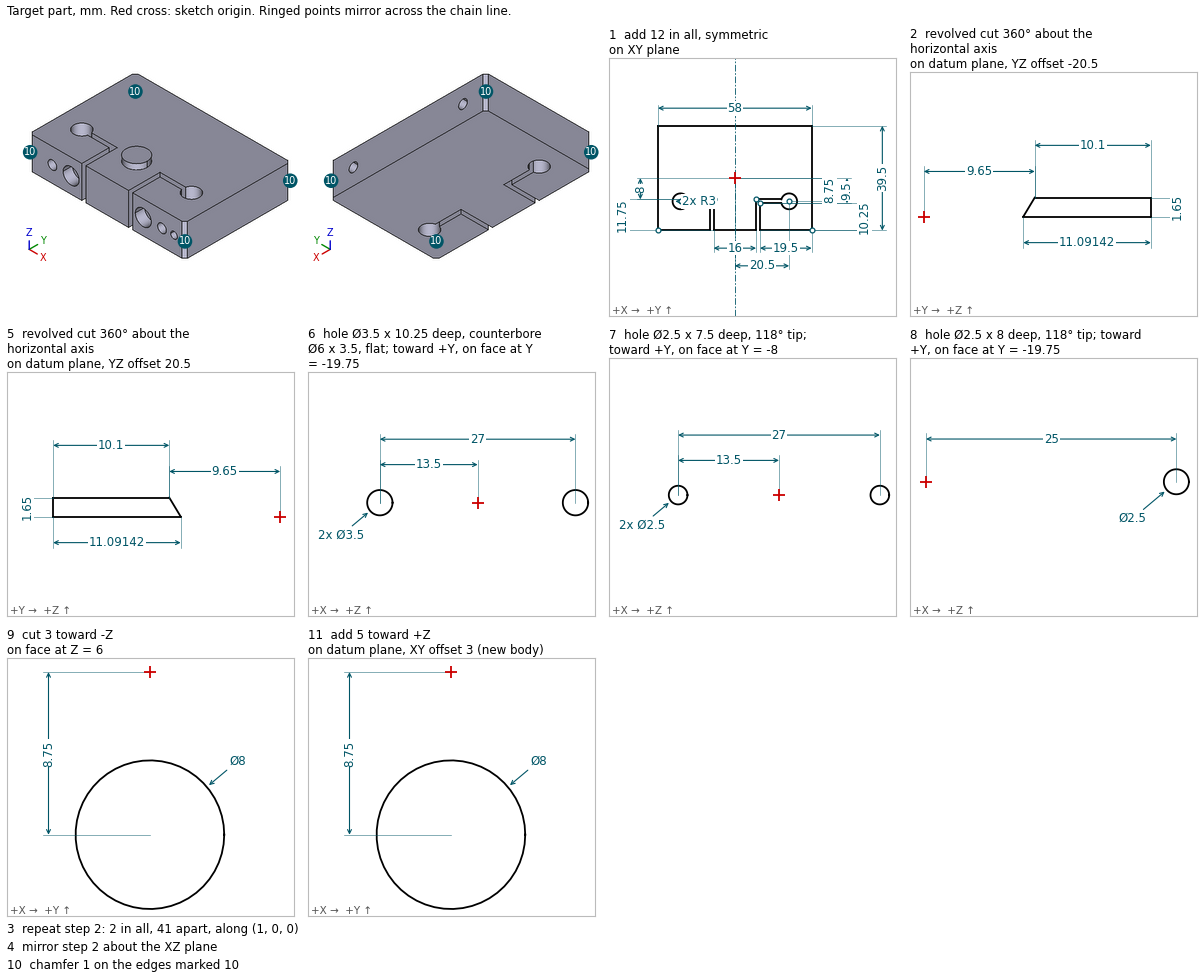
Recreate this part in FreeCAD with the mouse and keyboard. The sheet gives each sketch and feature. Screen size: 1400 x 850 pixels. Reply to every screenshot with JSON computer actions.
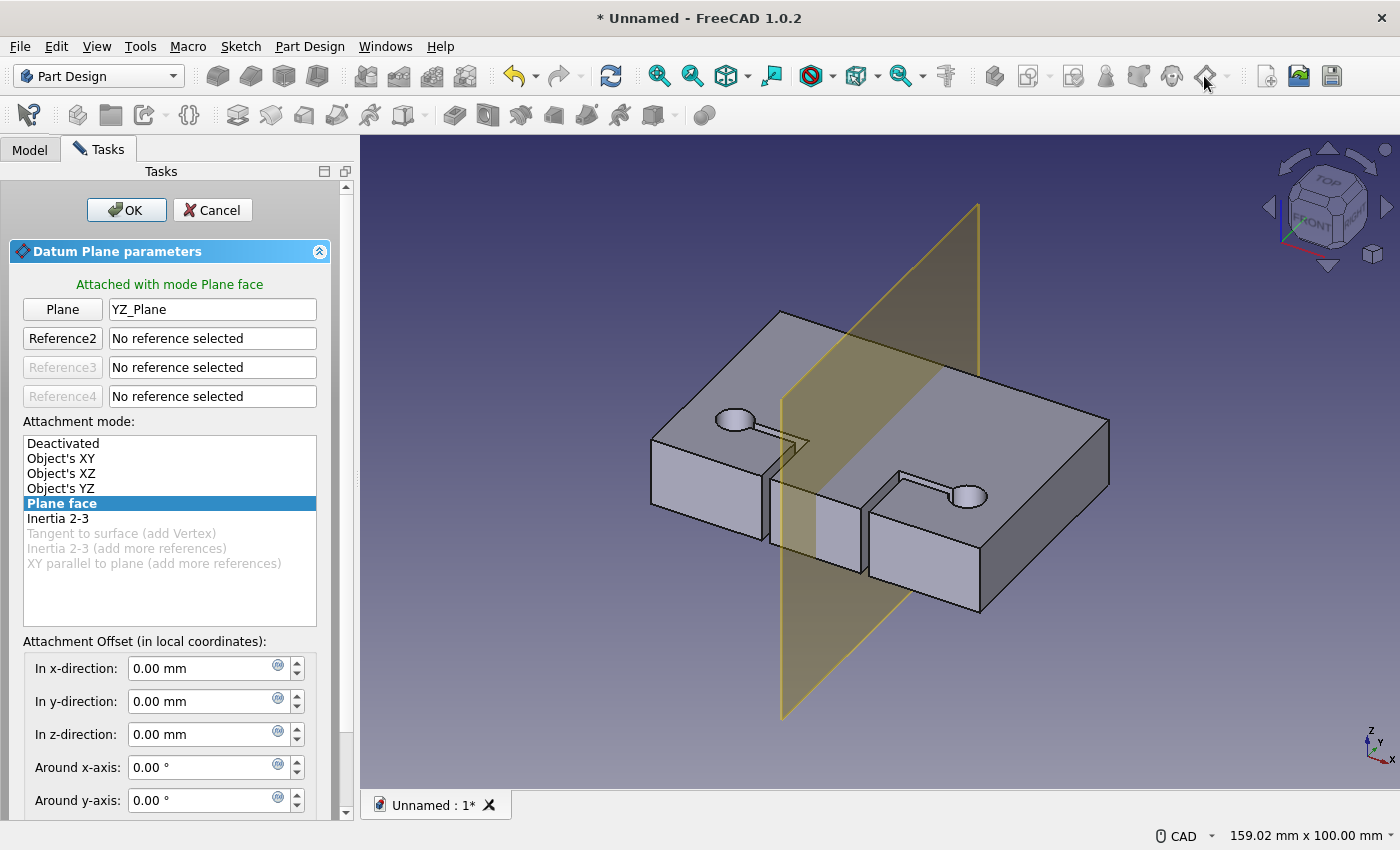
{"action": "triple_click", "coordinate": [210, 734]}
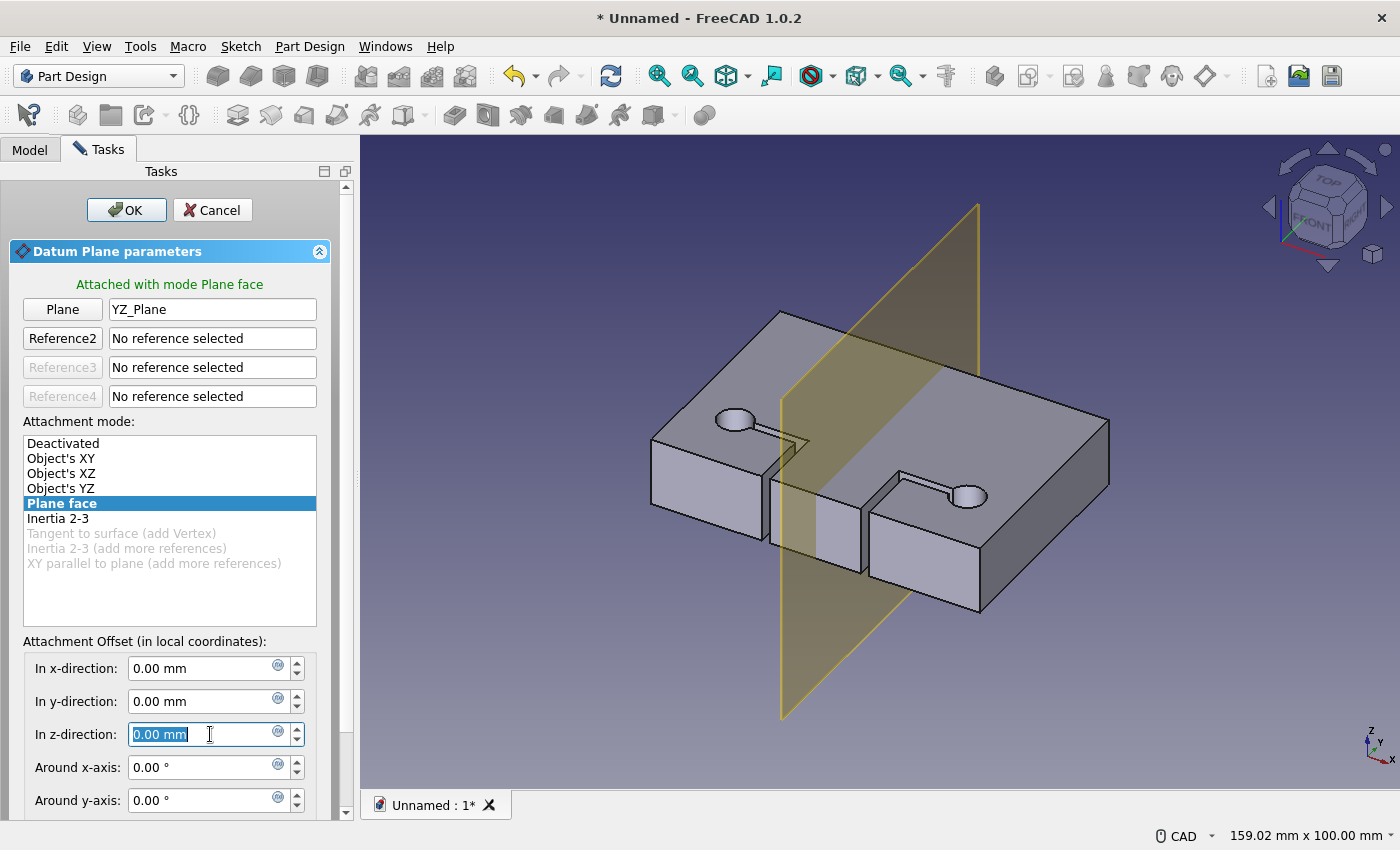
{"action": "type", "text": "-20.5"}
{"action": "key", "text": "Tab"}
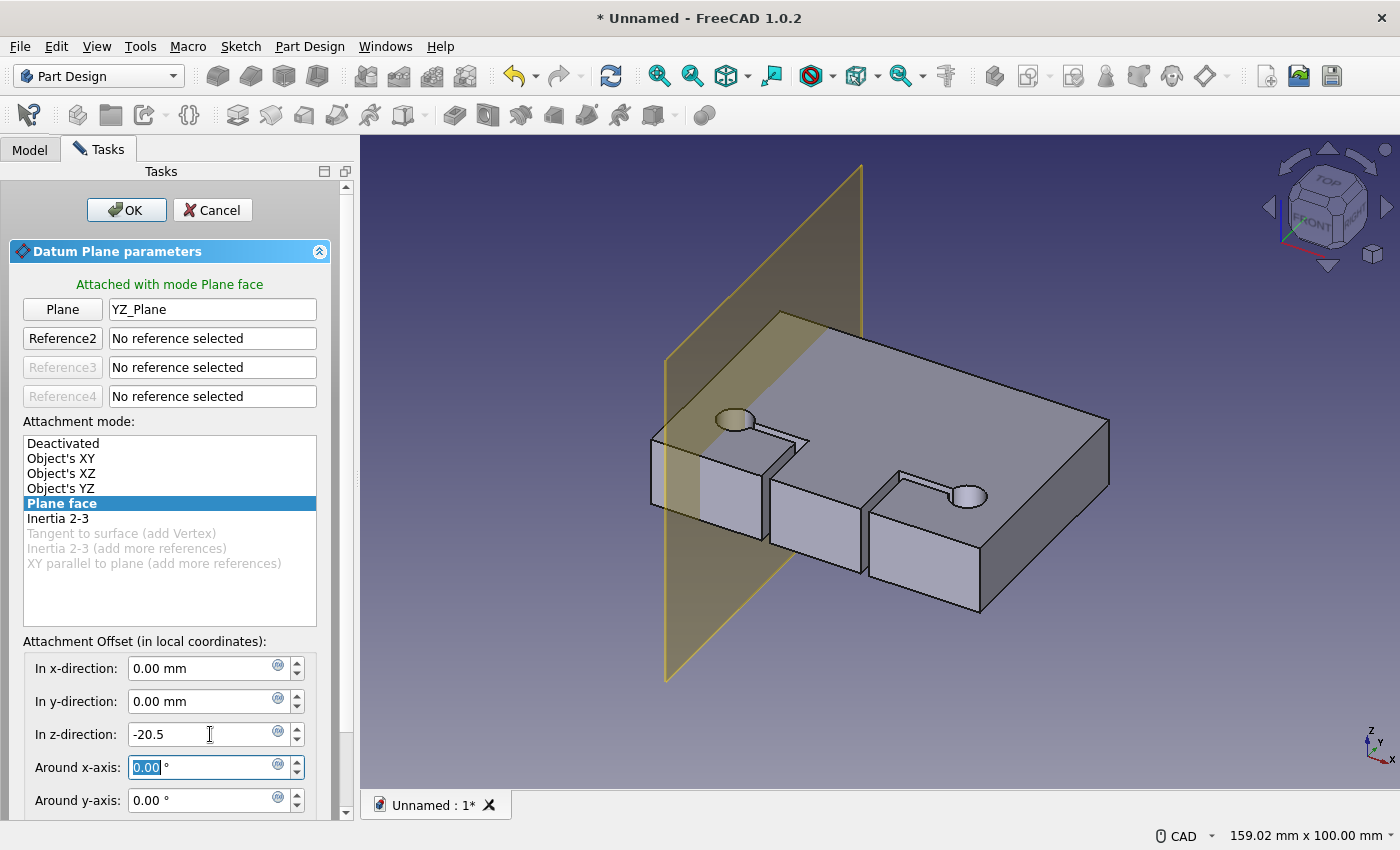
{"action": "left_click", "coordinate": [127, 210]}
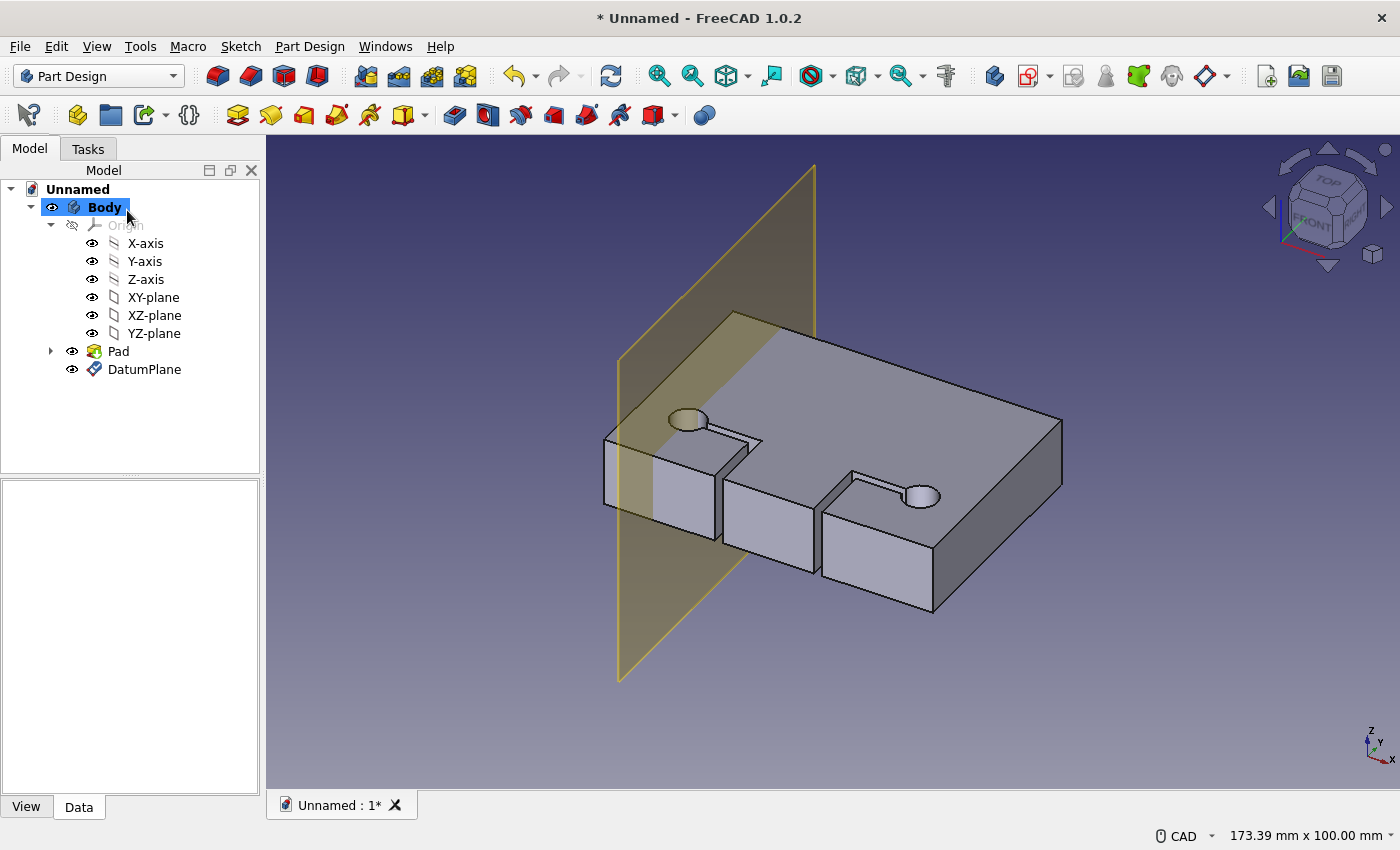
{"action": "left_click", "coordinate": [117, 369]}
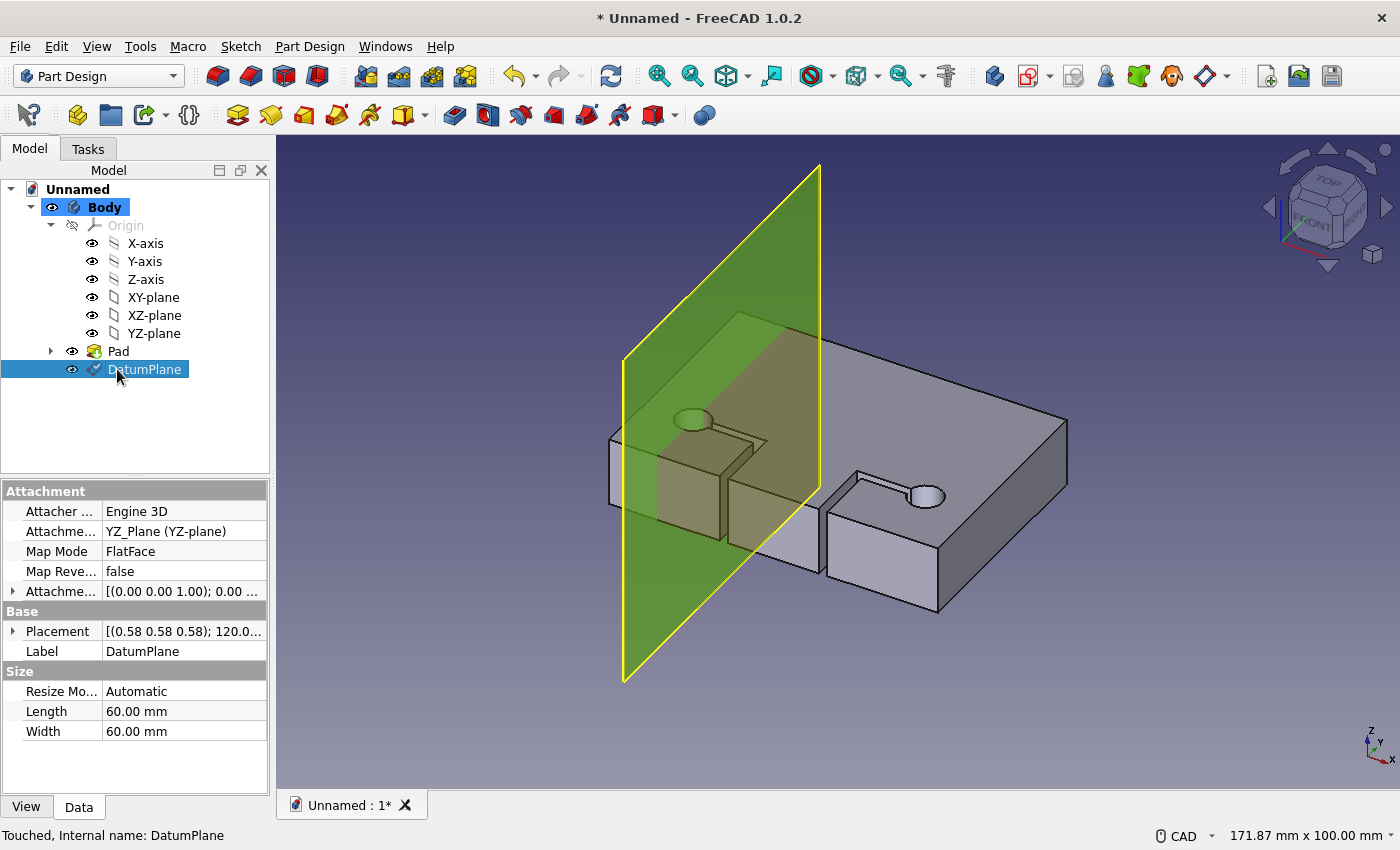
{"action": "left_click", "coordinate": [1028, 76]}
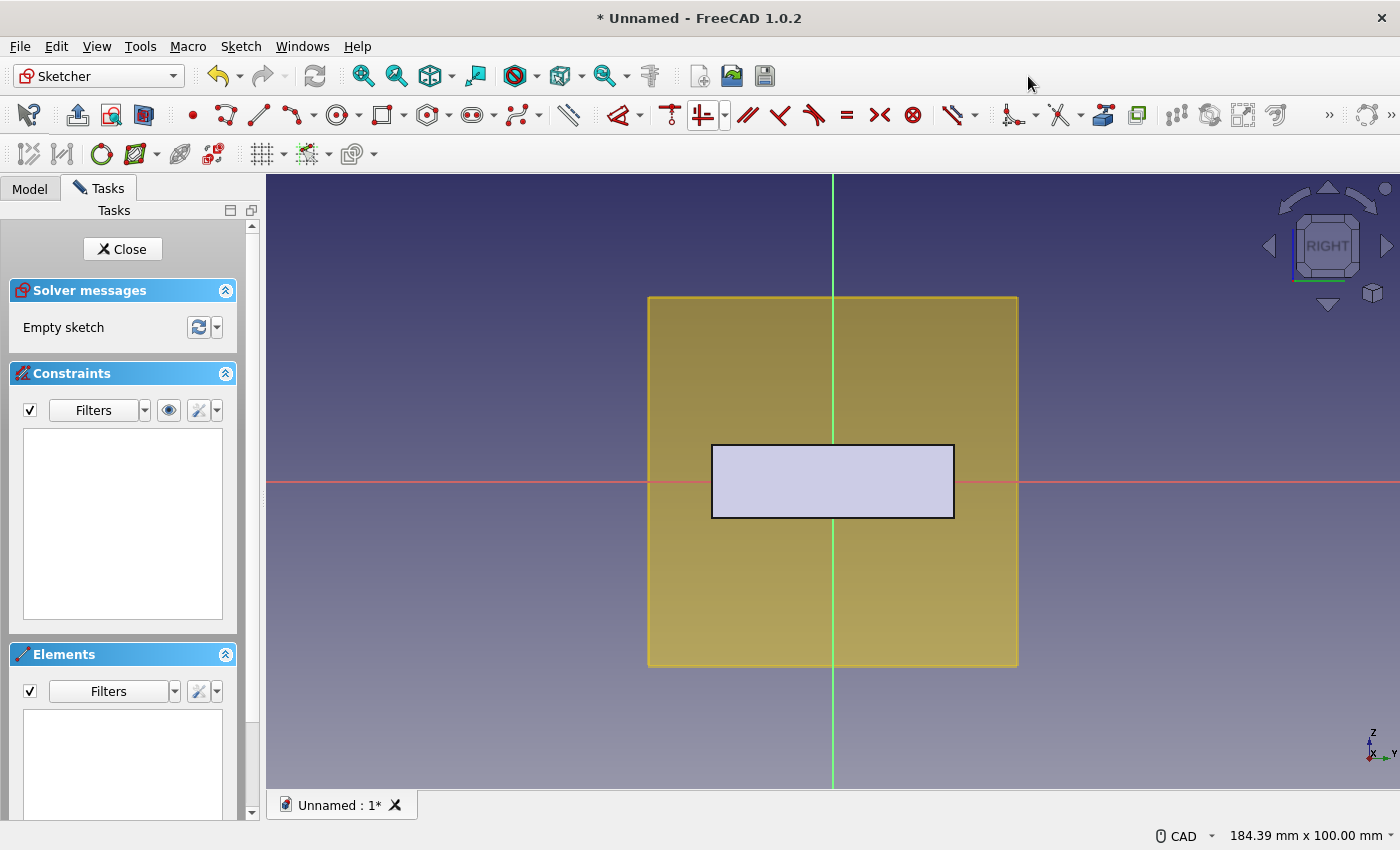
{"action": "key", "text": "q s"}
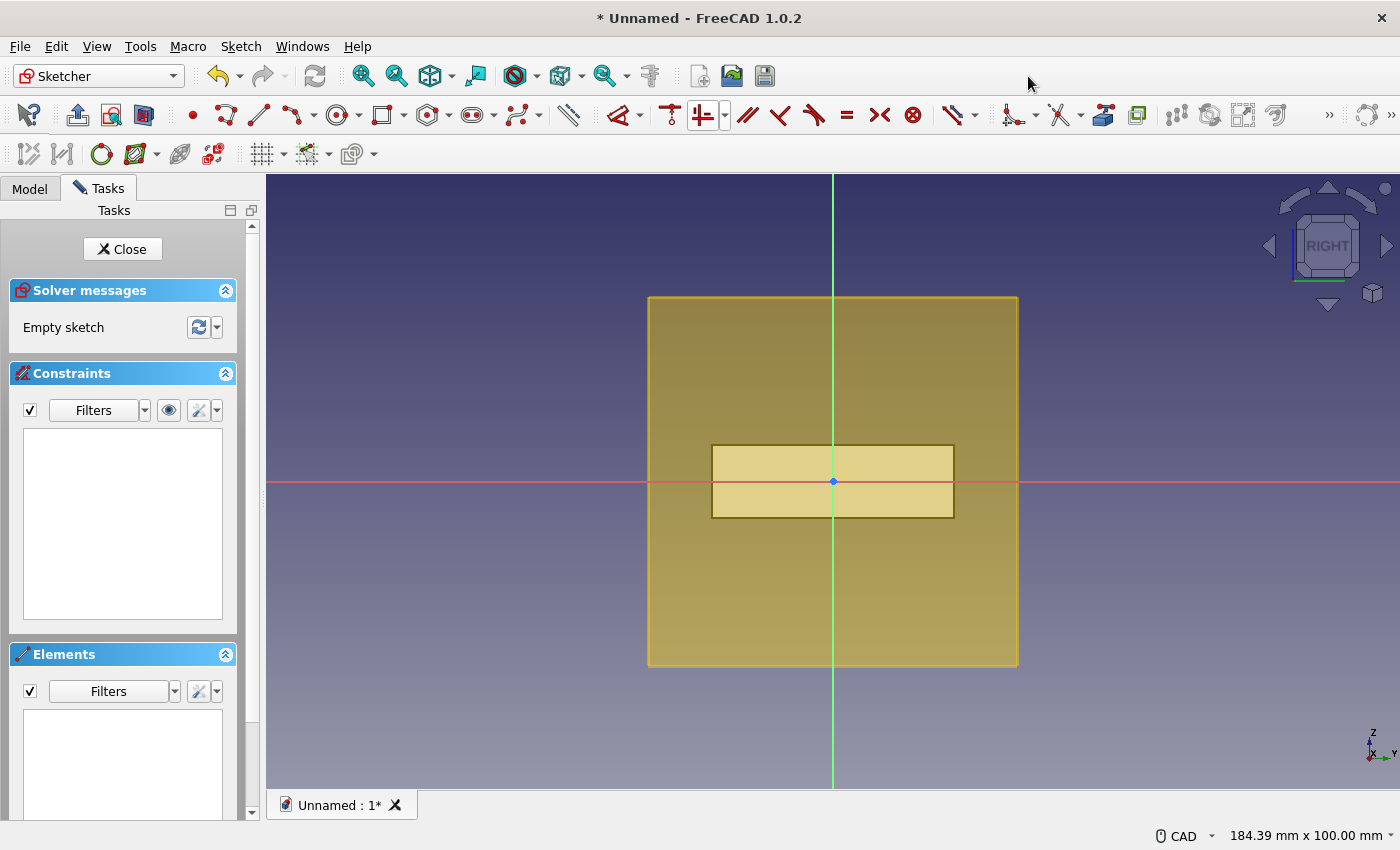
{"action": "scroll", "coordinate": [926, 475], "scroll_direction": "up", "scroll_amount": 8}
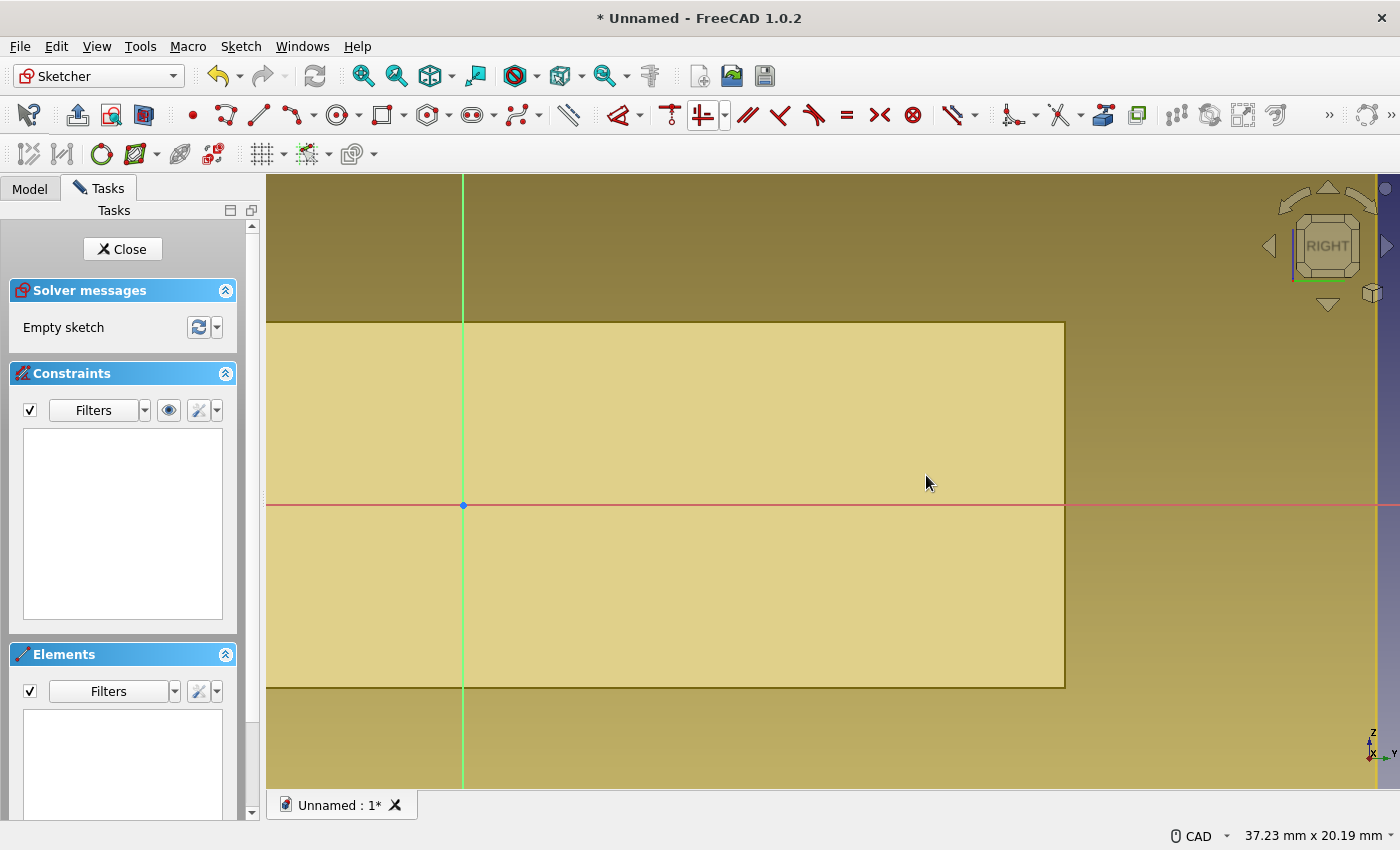
{"action": "key", "text": "g m"}